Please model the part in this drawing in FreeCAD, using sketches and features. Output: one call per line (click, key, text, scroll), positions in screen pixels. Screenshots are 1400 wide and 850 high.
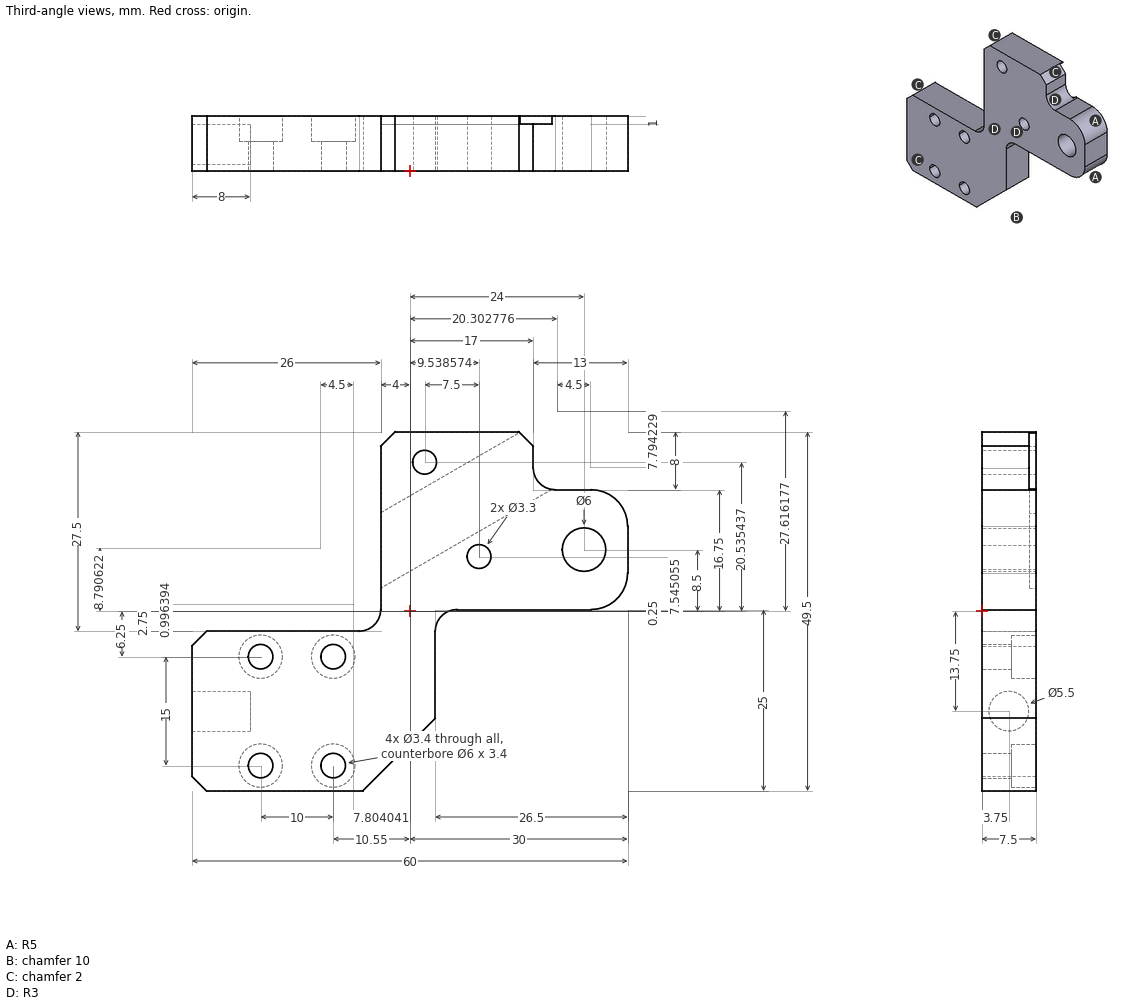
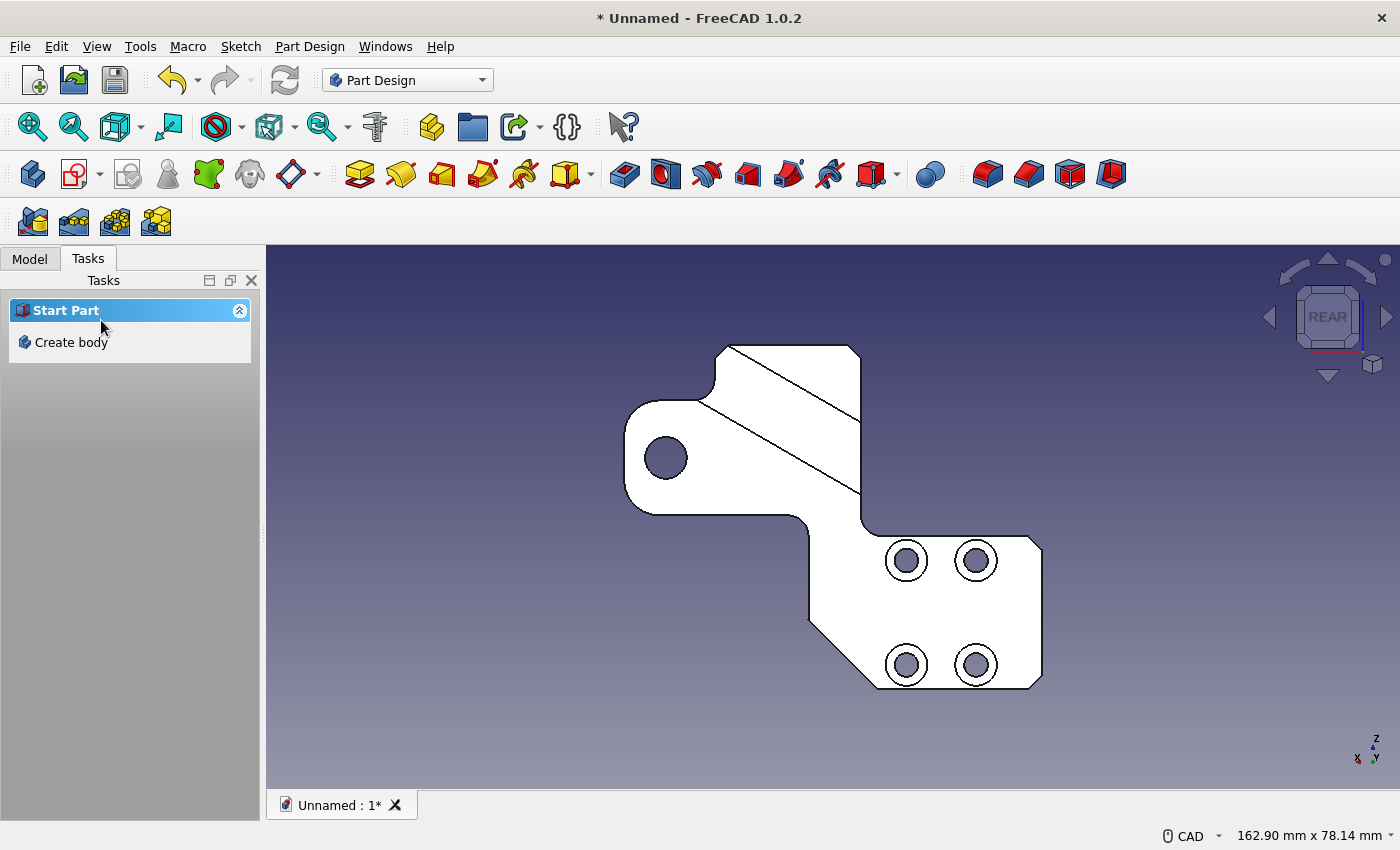
click(1012, 626)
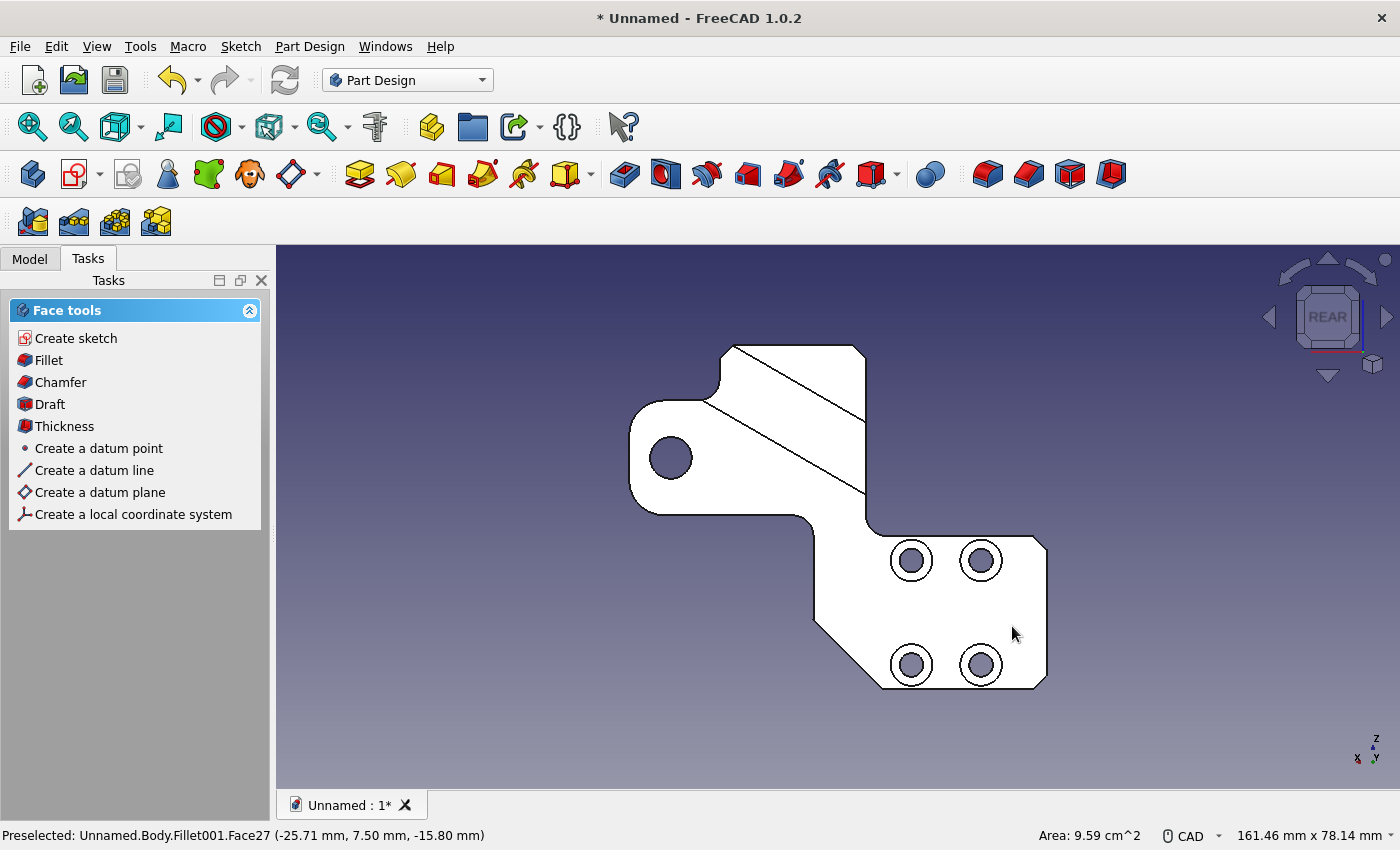
click(74, 174)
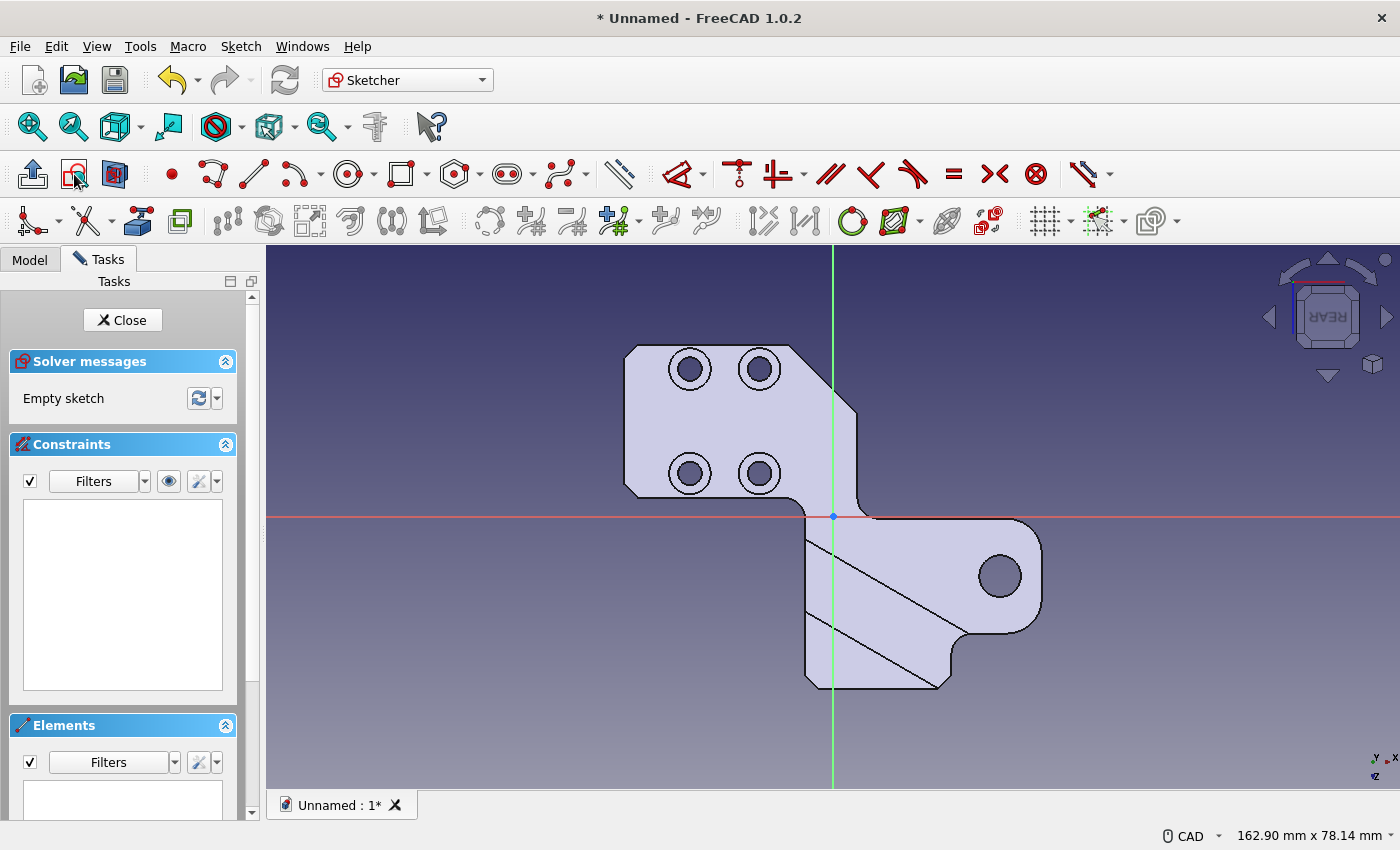
scroll(960, 657, up, 4)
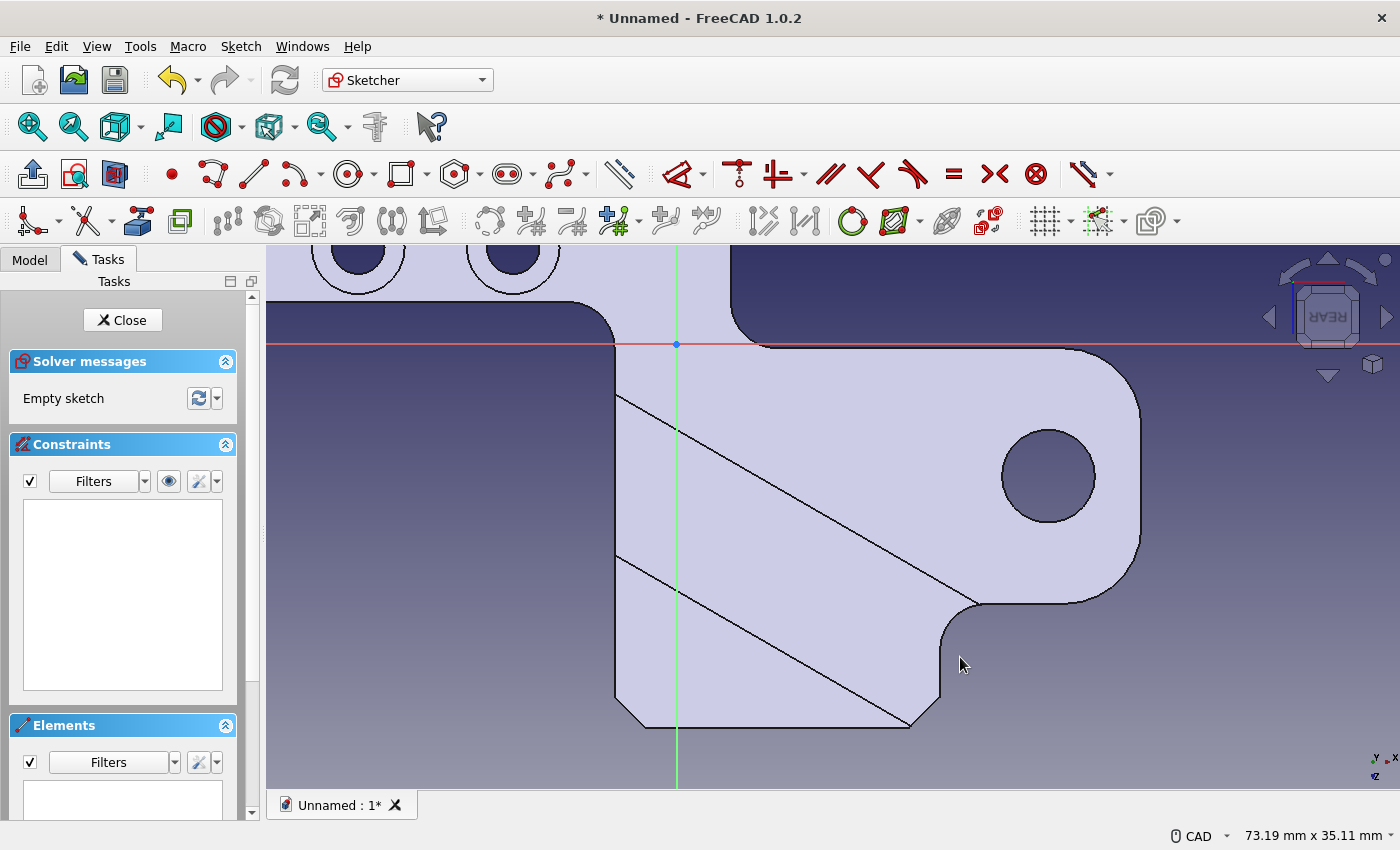
key(g)
key(c)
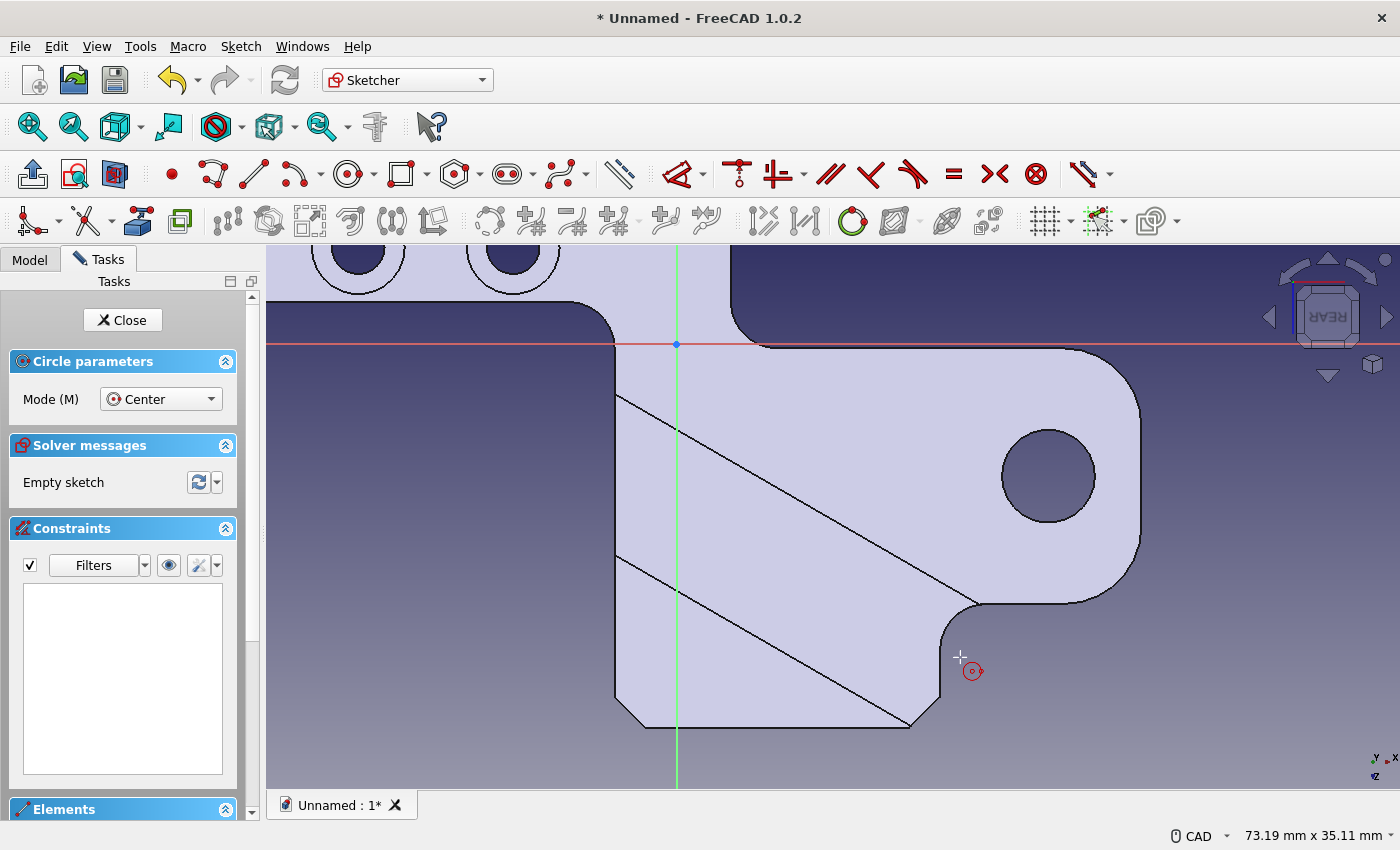
click(824, 461)
move(842, 443)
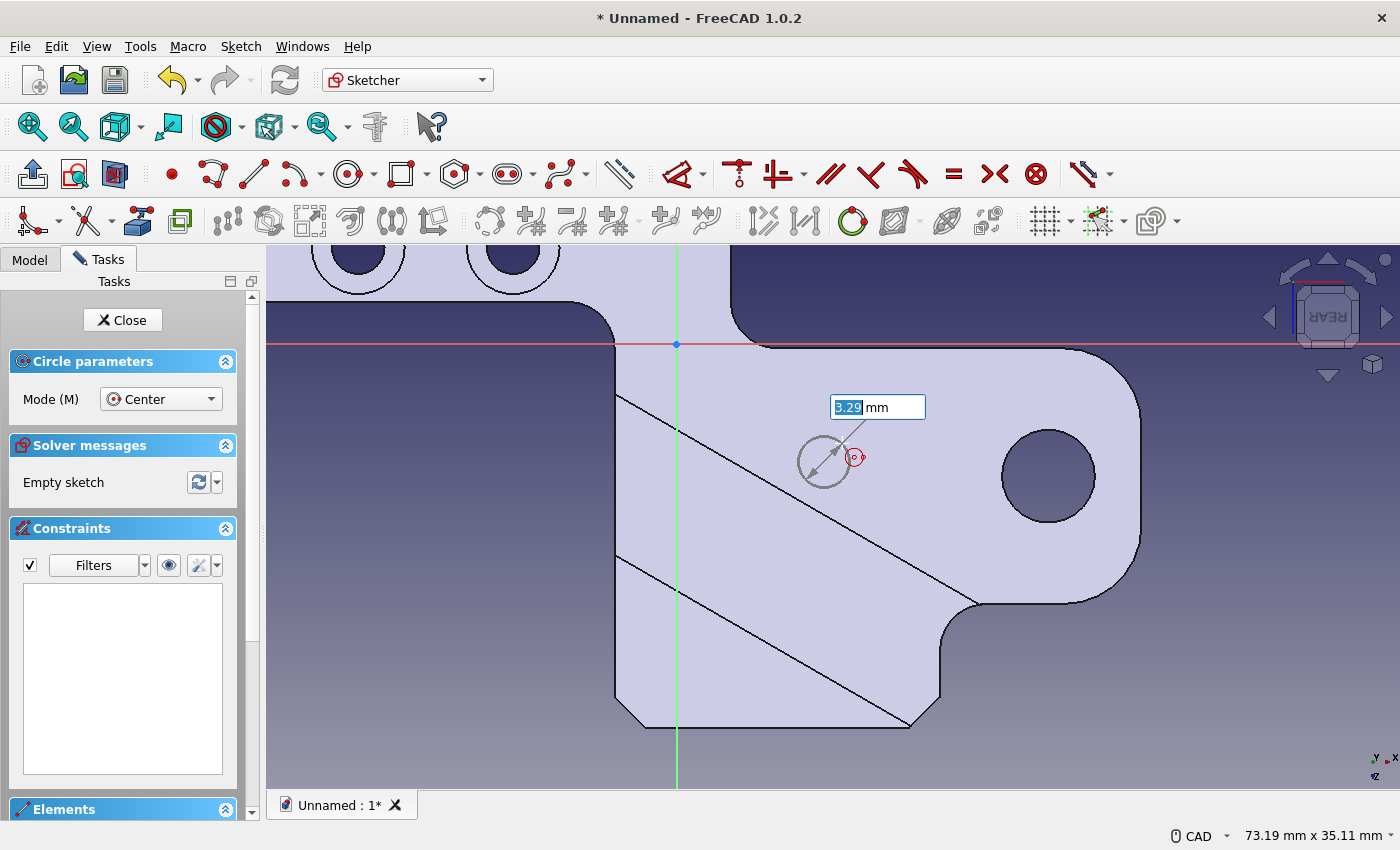
text(3.3)
key(Return)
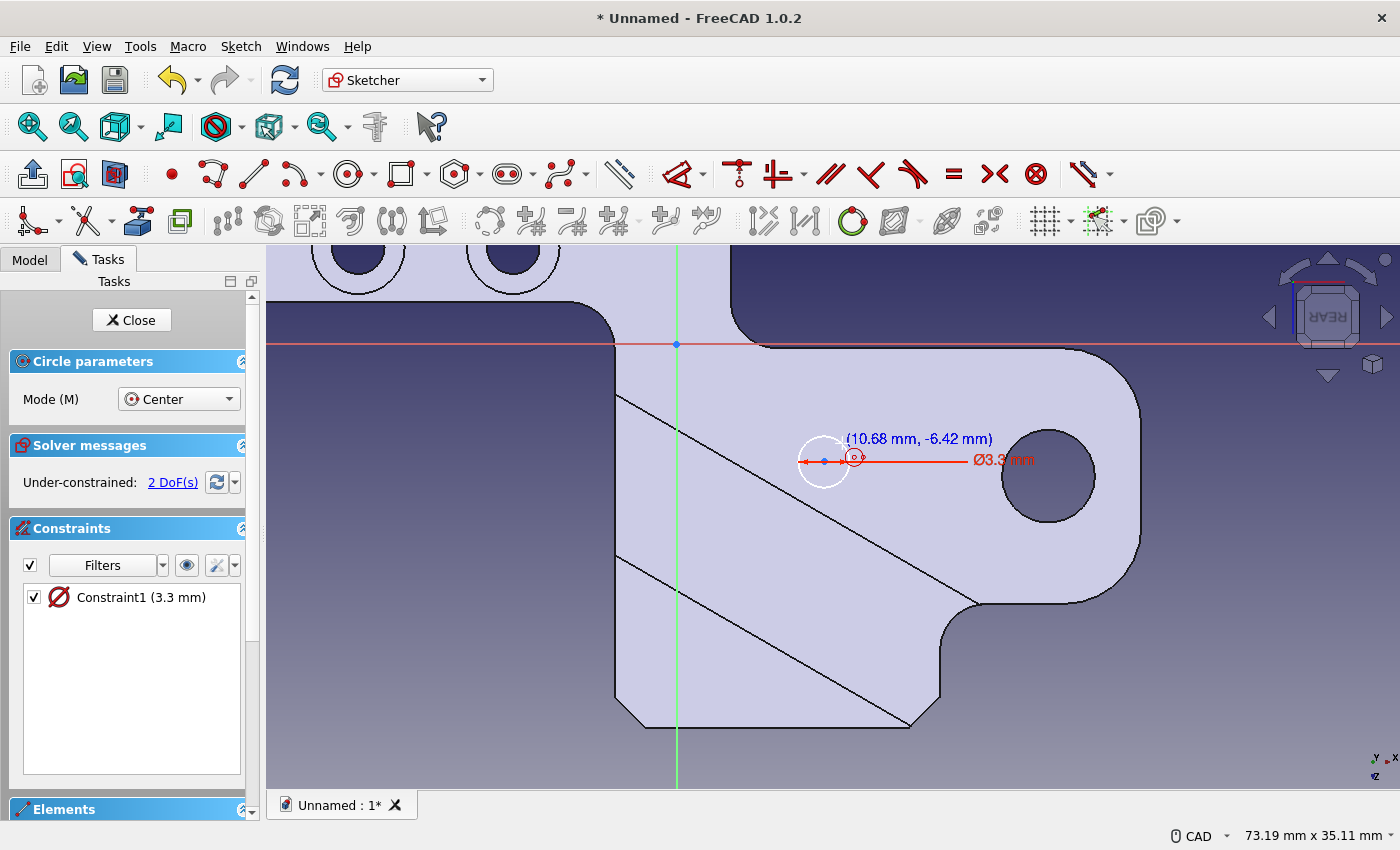
click(708, 663)
move(726, 645)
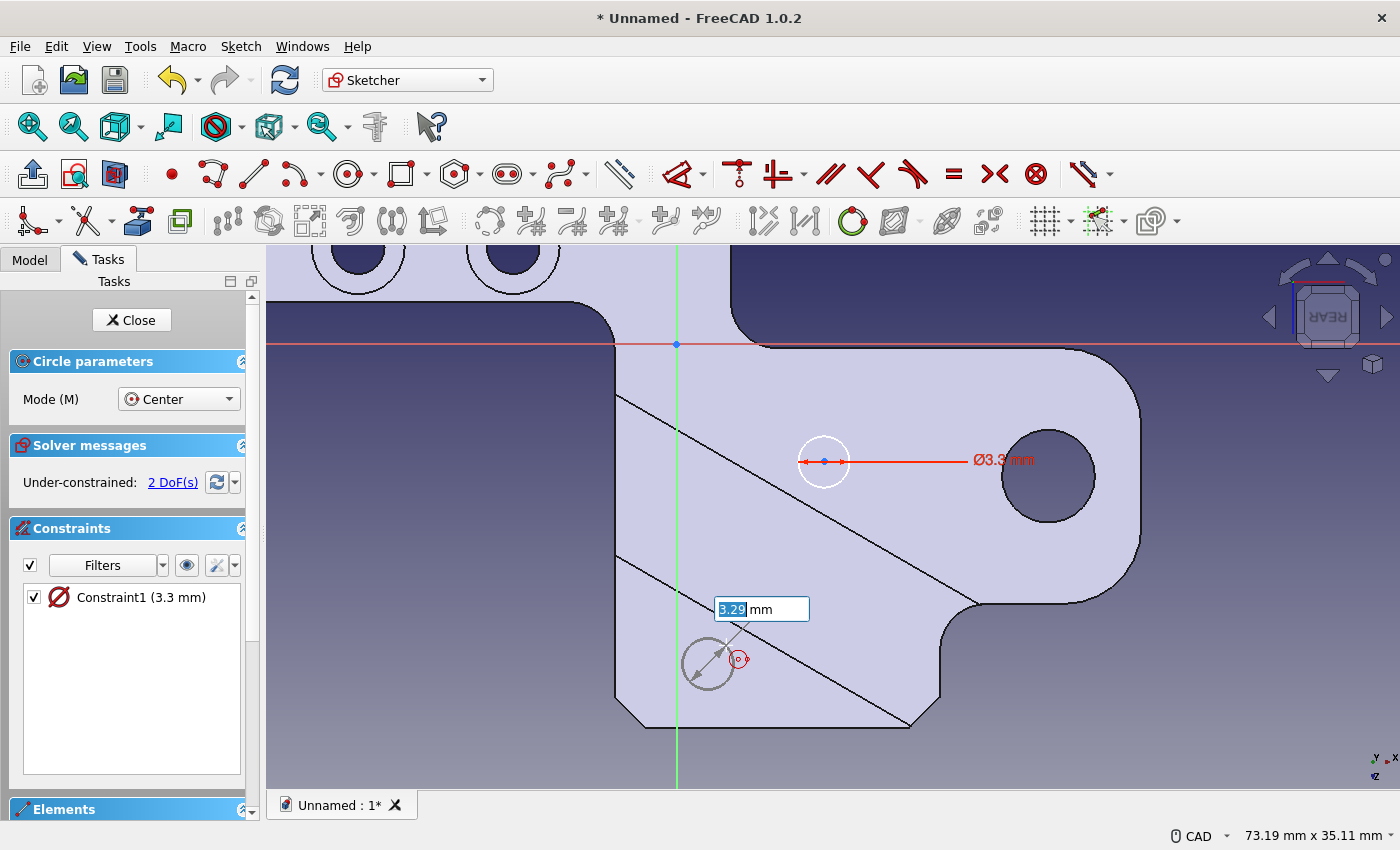
text(3.3)
key(Return)
key(Escape)